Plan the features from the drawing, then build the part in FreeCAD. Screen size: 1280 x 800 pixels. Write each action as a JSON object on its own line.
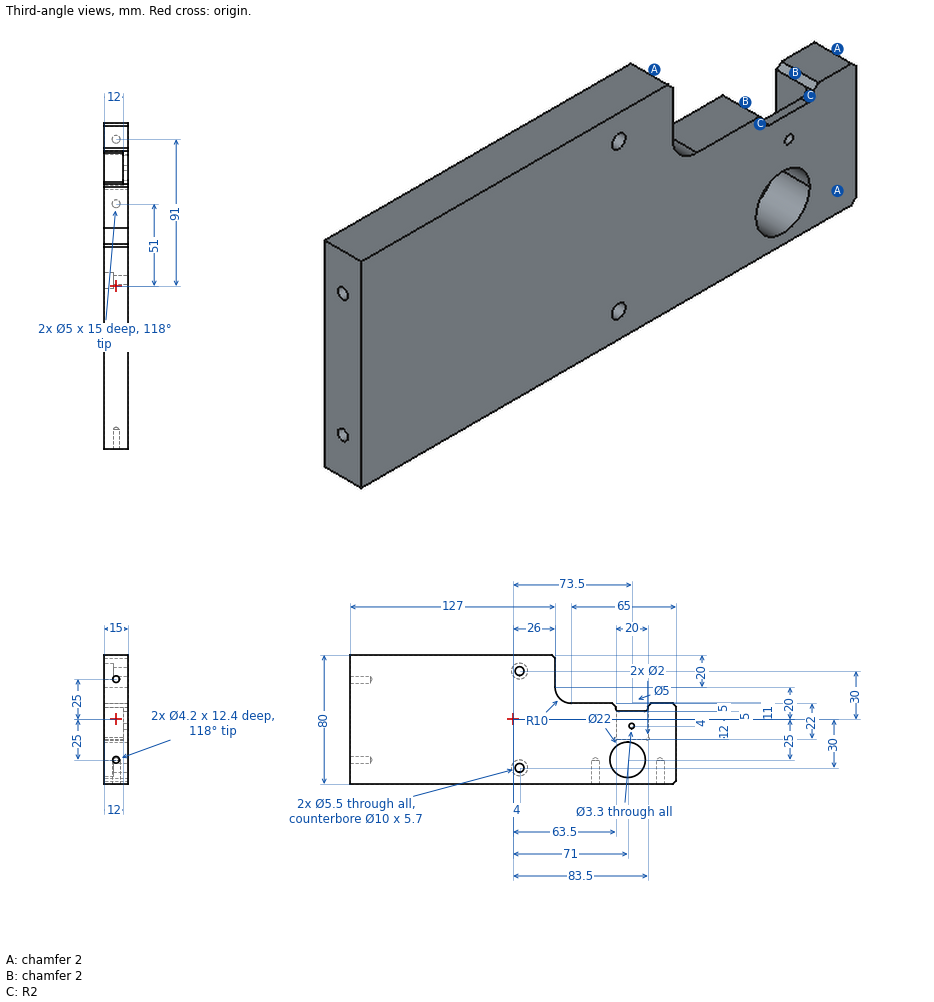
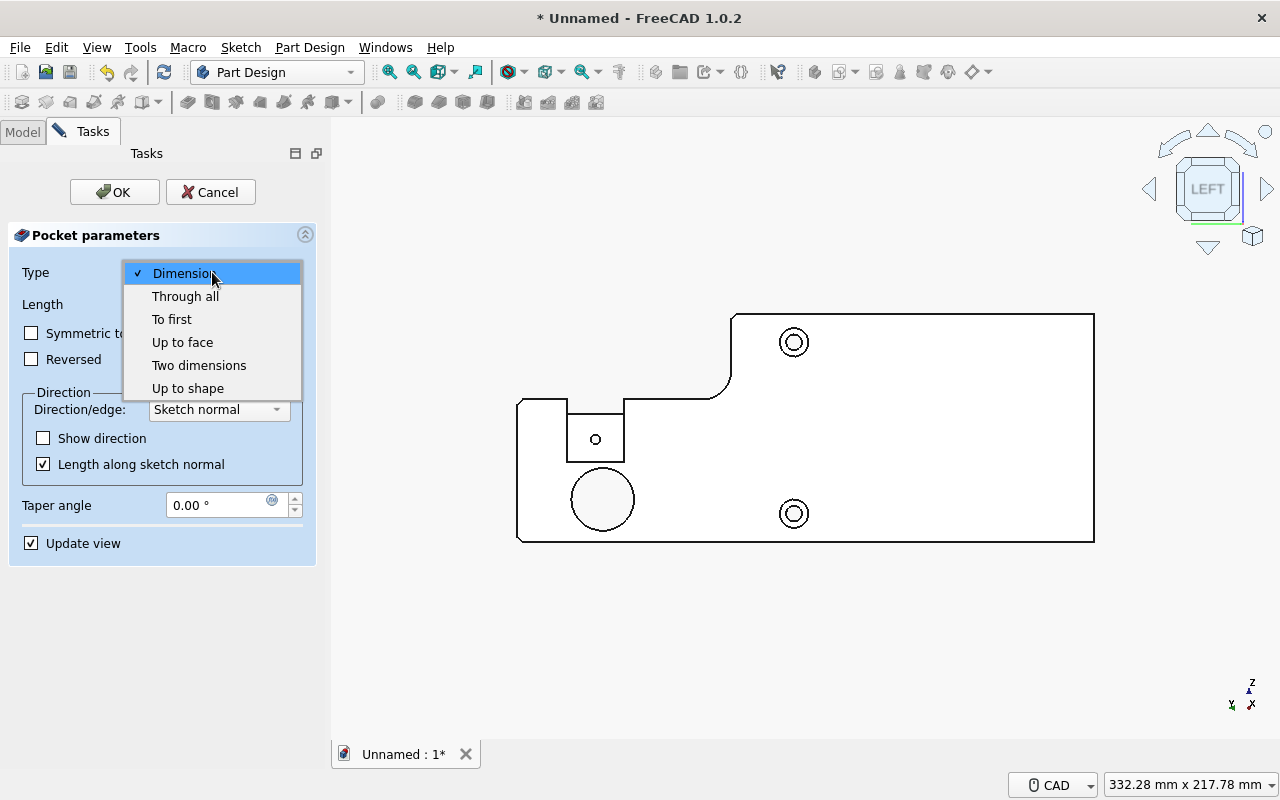
{"action": "left_click", "coordinate": [212, 296]}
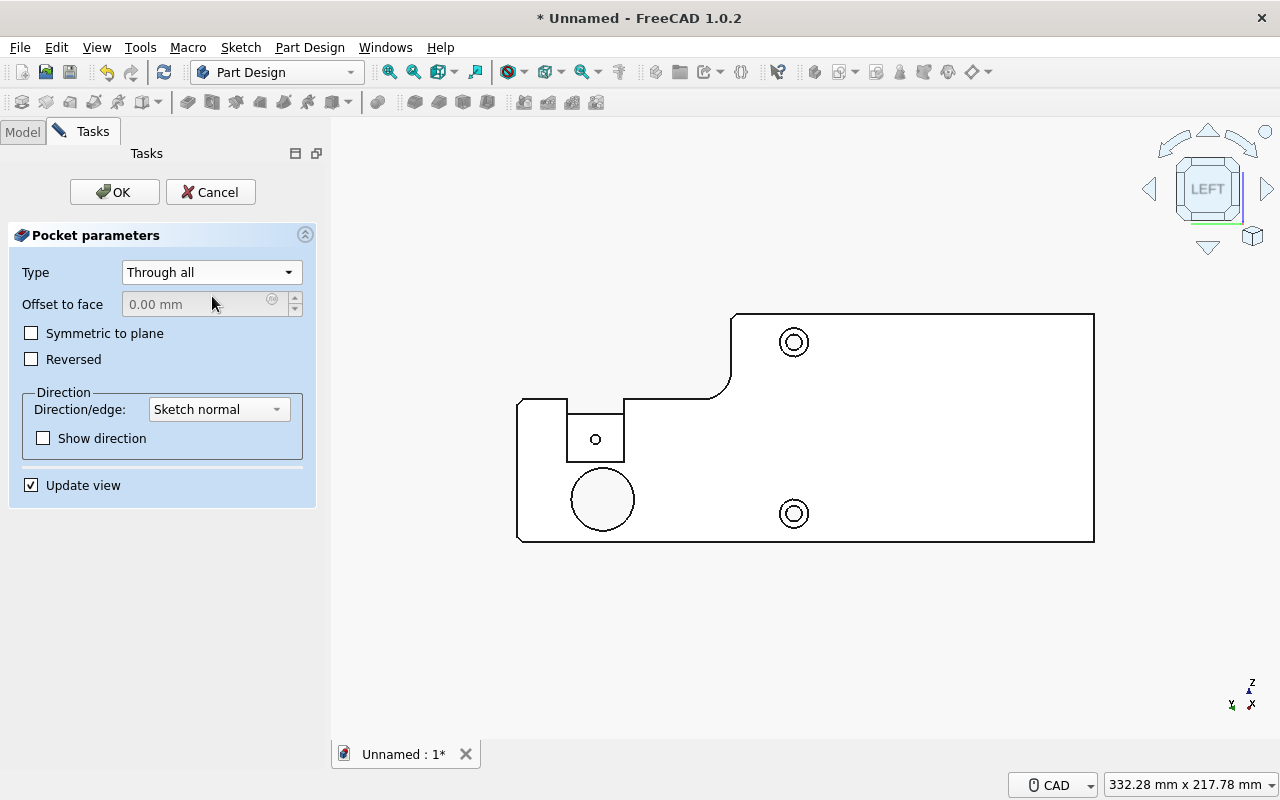
{"action": "left_click", "coordinate": [115, 192]}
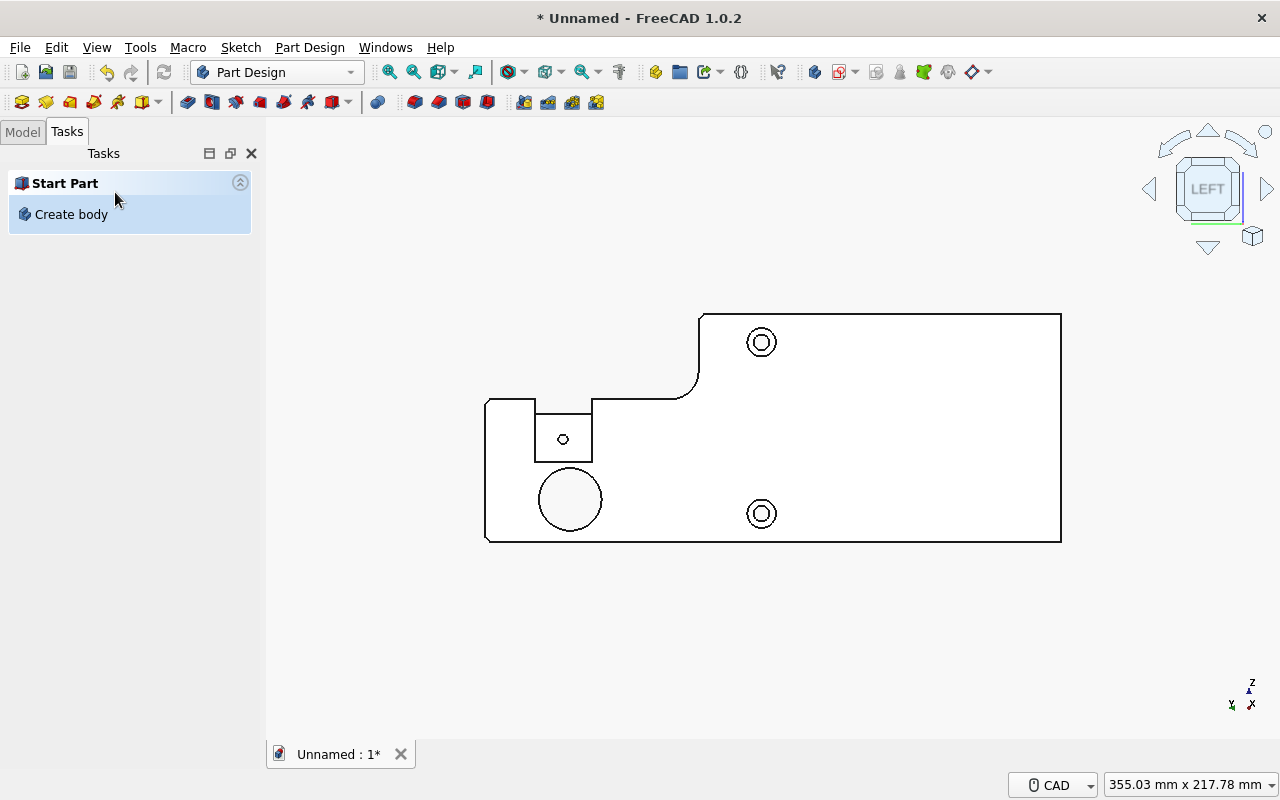
{"action": "left_click", "coordinate": [938, 427]}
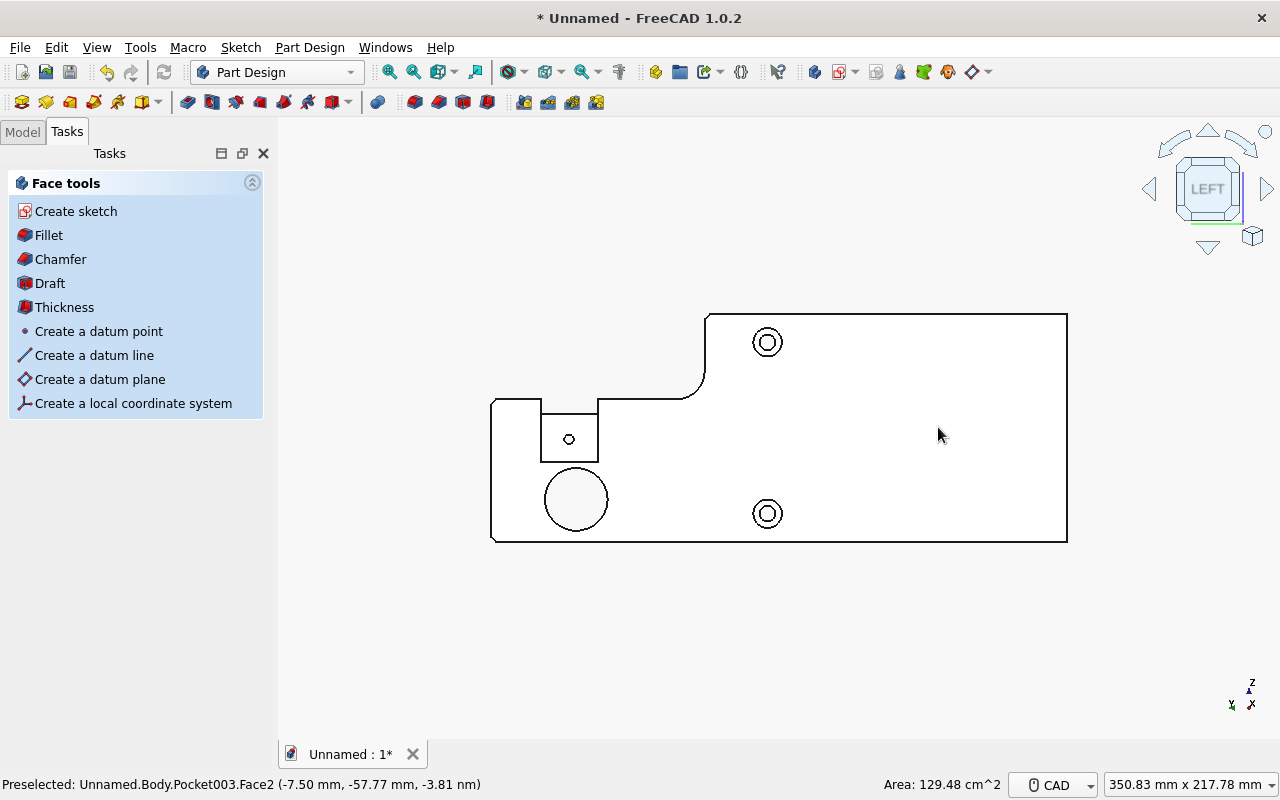
{"action": "left_click", "coordinate": [840, 72]}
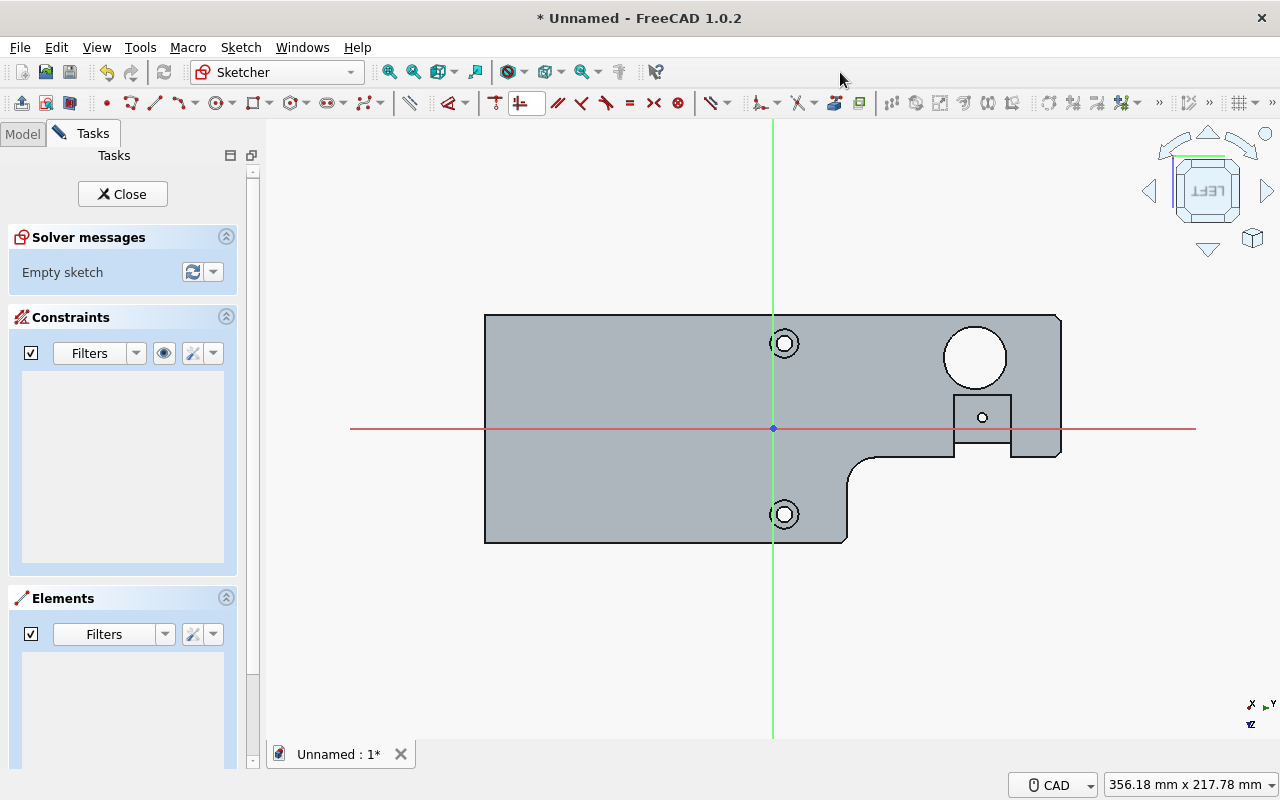
{"action": "scroll", "coordinate": [1017, 391], "scroll_direction": "up", "scroll_amount": 11}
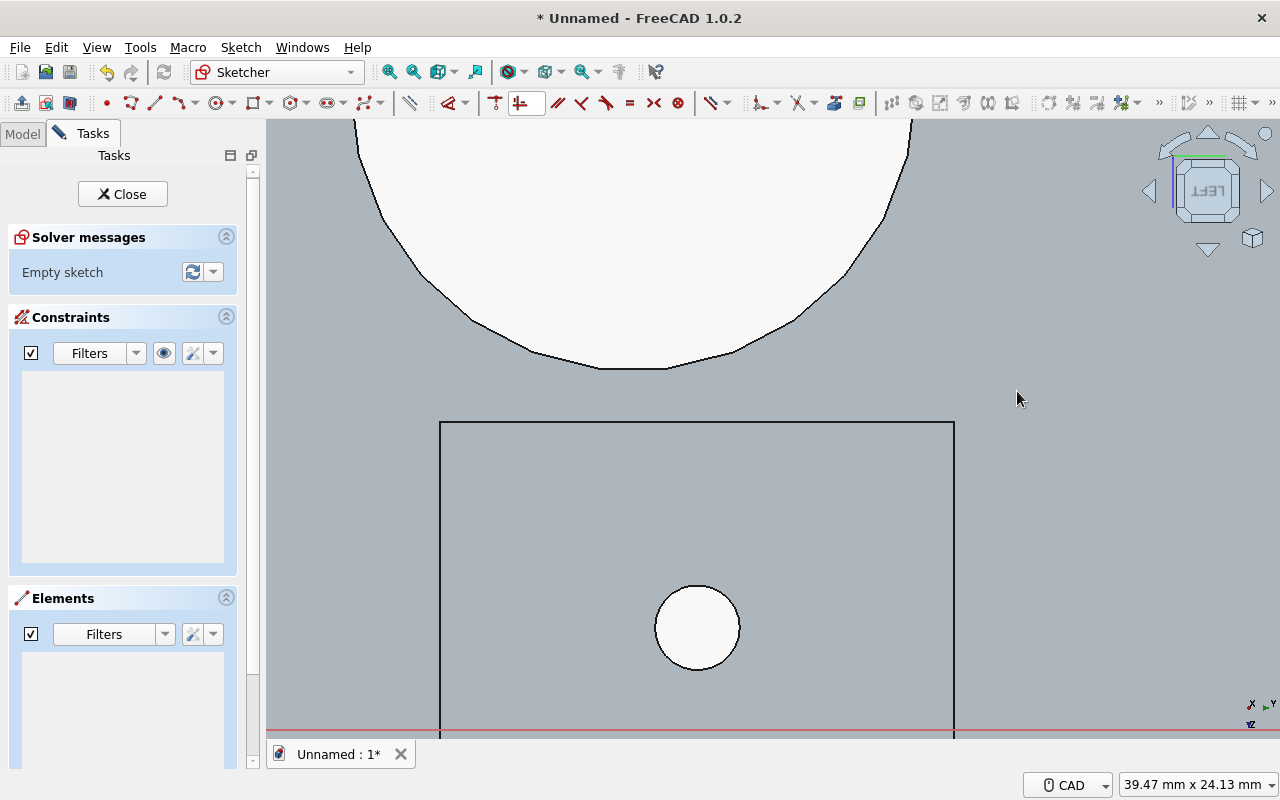
{"action": "left_click", "coordinate": [216, 104]}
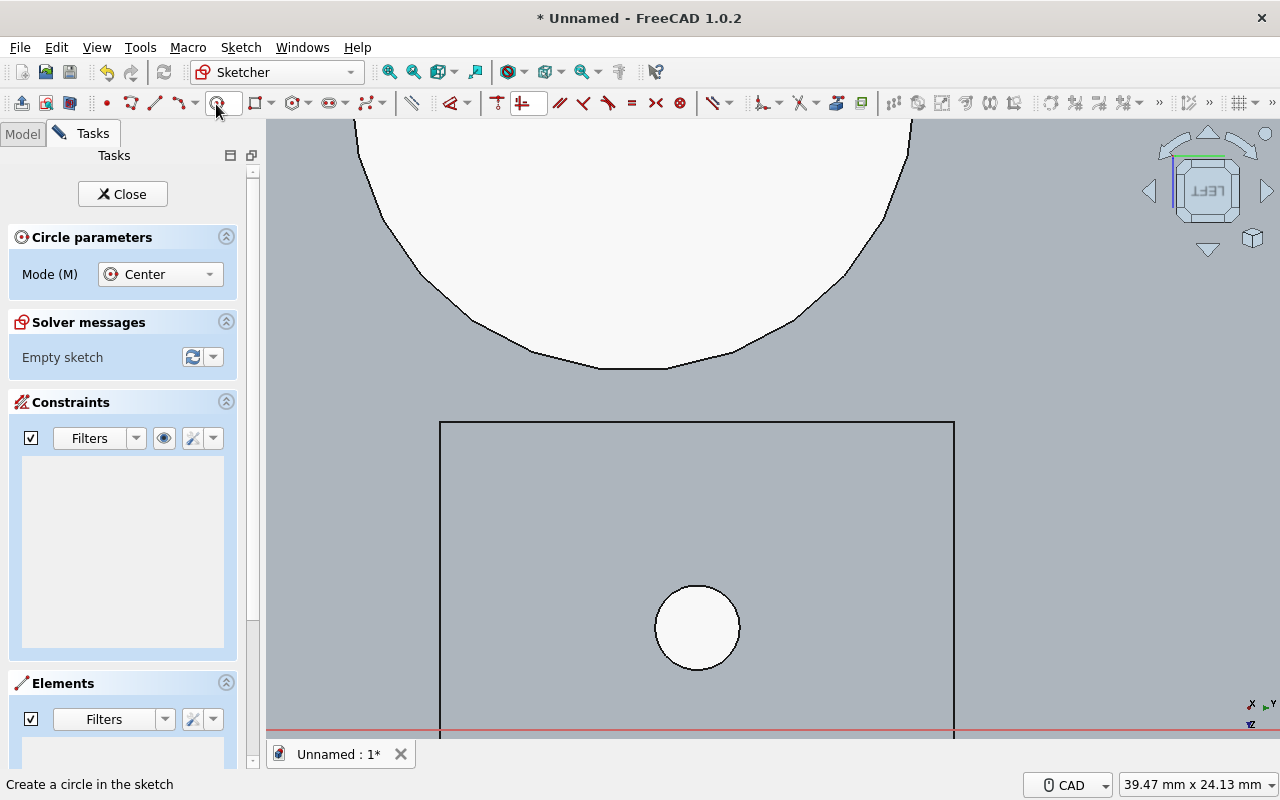
{"action": "left_click", "coordinate": [954, 422]}
{"action": "left_click", "coordinate": [972, 404]}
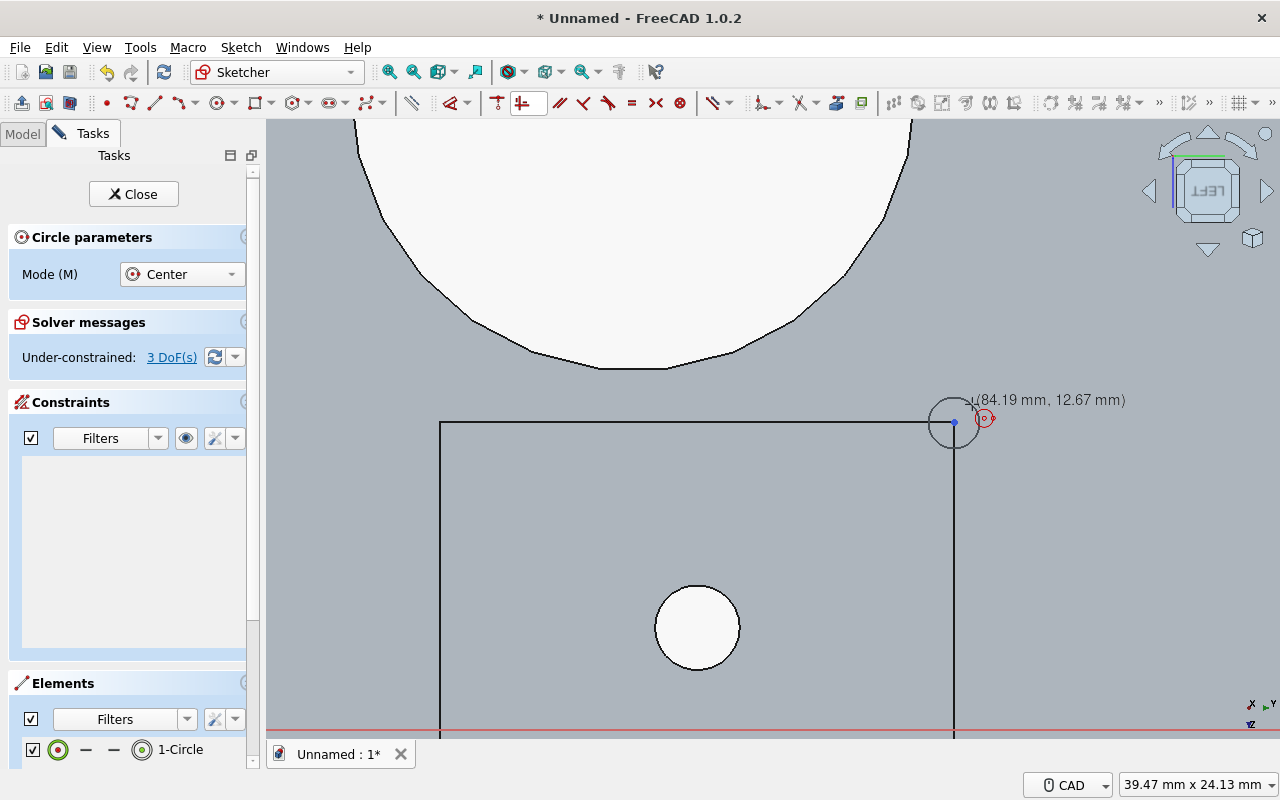
{"action": "left_click", "coordinate": [440, 422]}
{"action": "left_click", "coordinate": [459, 404]}
{"action": "key", "text": "Escape"}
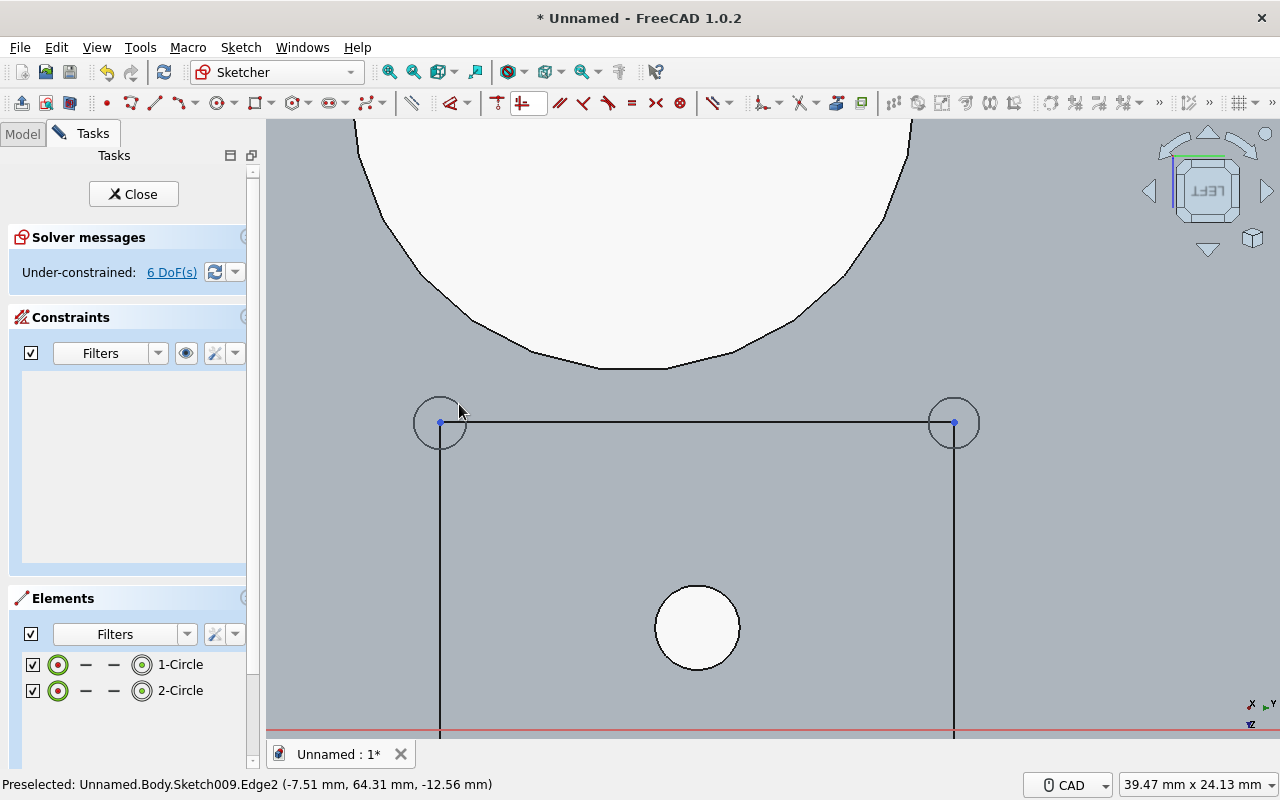
{"action": "left_click", "coordinate": [972, 405]}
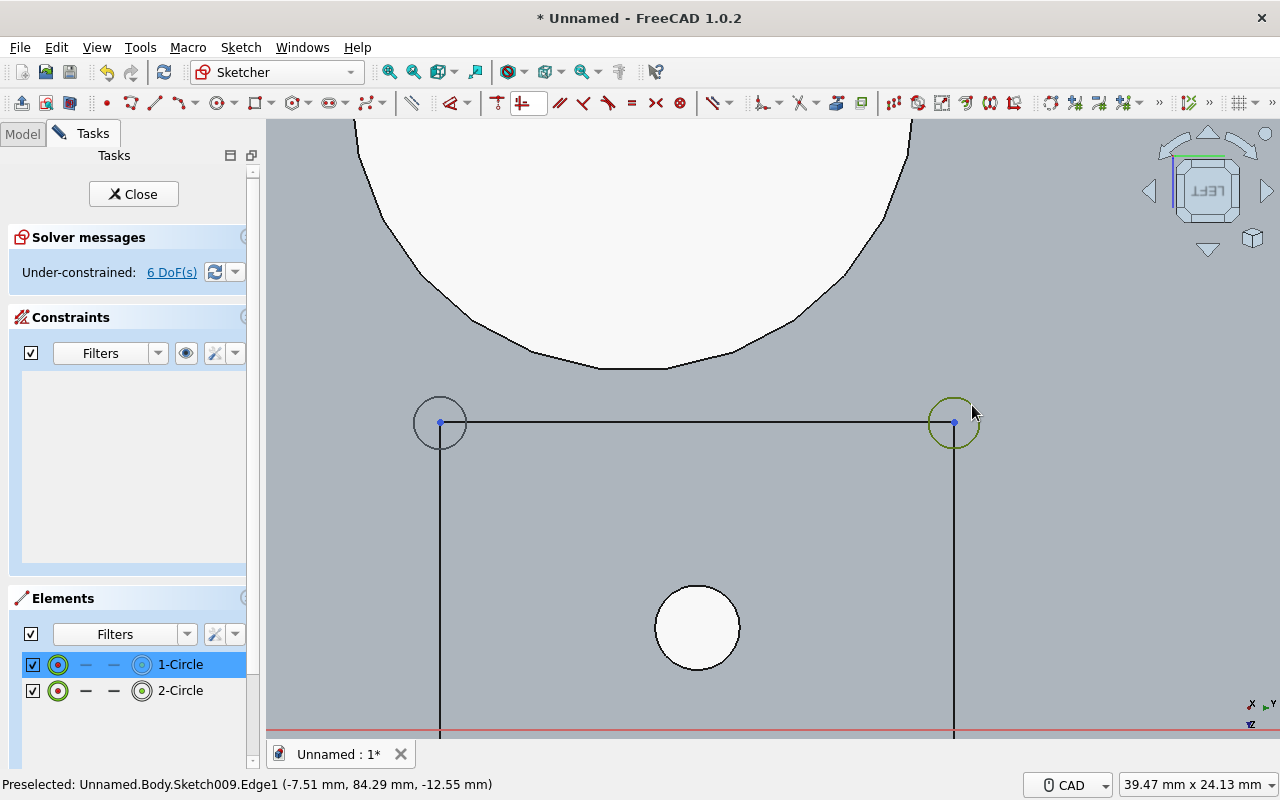
{"action": "left_click", "coordinate": [458, 404]}